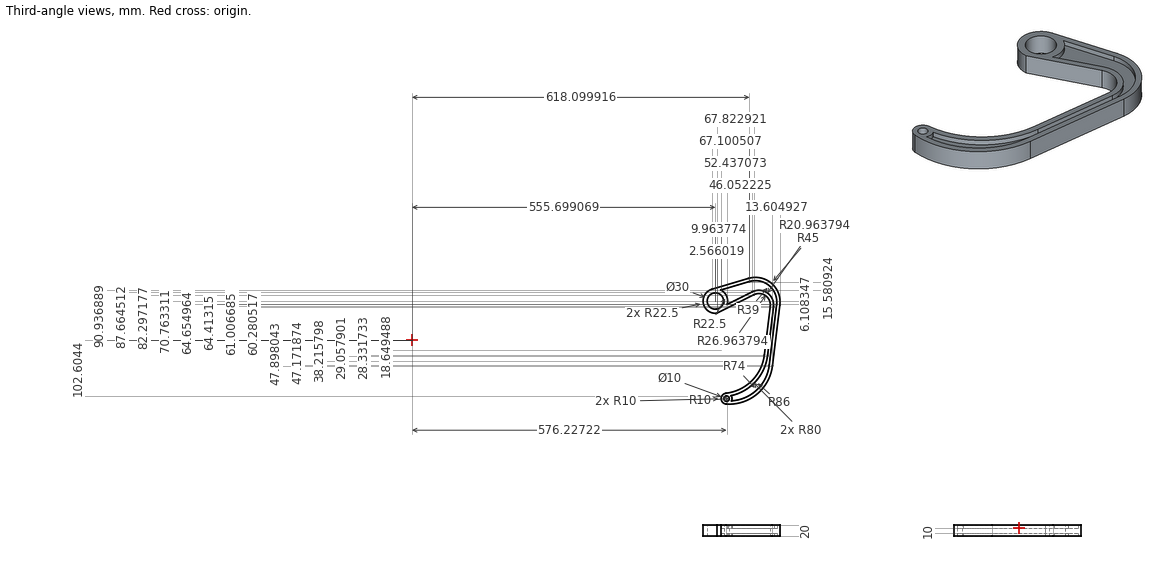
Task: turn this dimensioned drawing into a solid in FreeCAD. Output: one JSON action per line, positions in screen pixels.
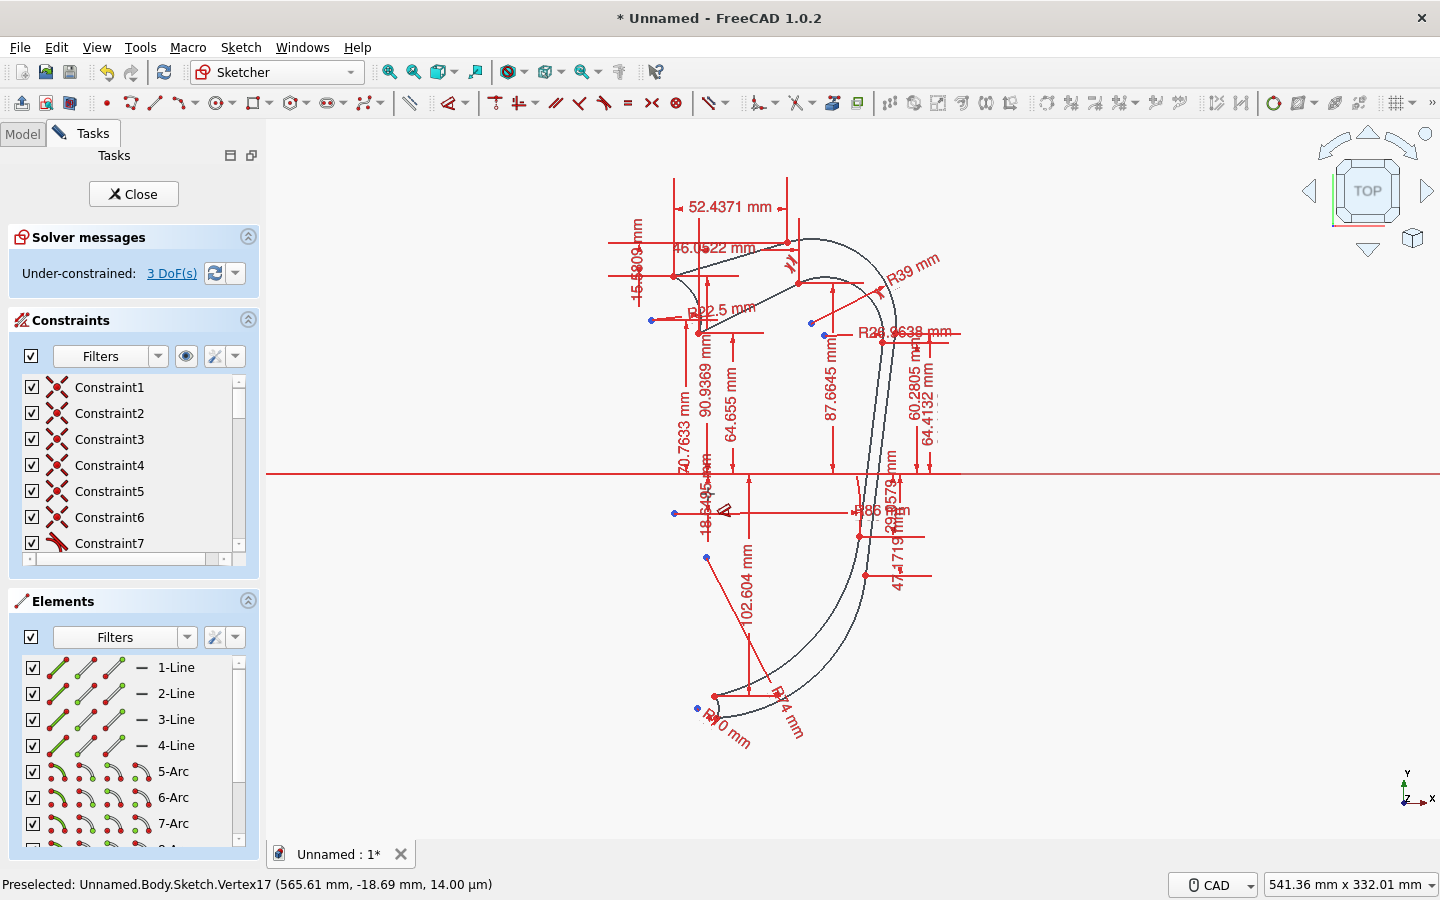
{"action": "left_click", "coordinate": [697, 709]}
{"action": "left_click", "coordinate": [496, 743]}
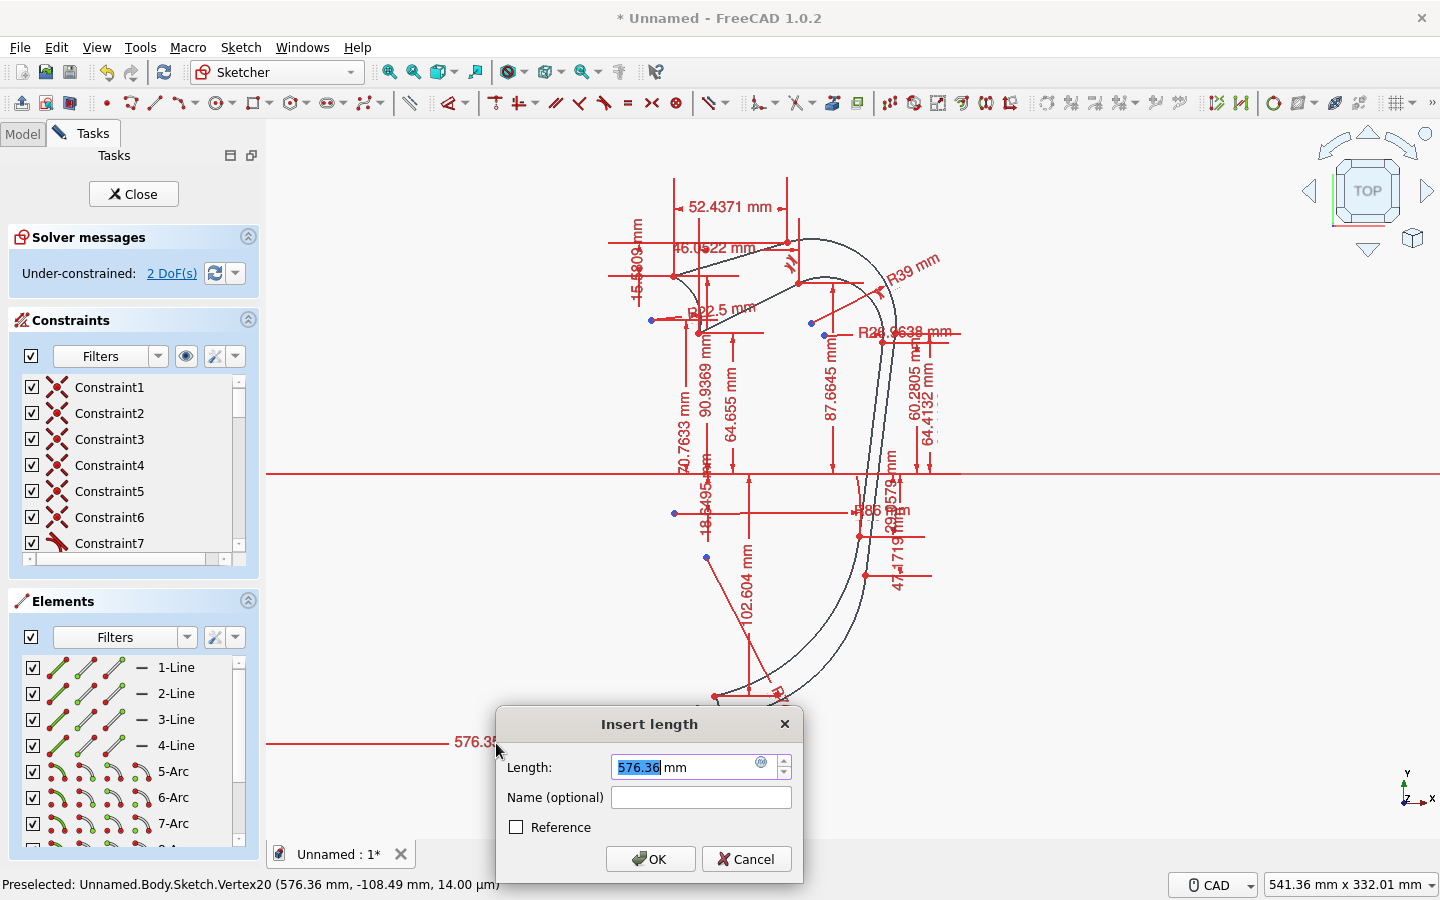
{"action": "type", "text": "576.22722"}
{"action": "key", "text": "Return"}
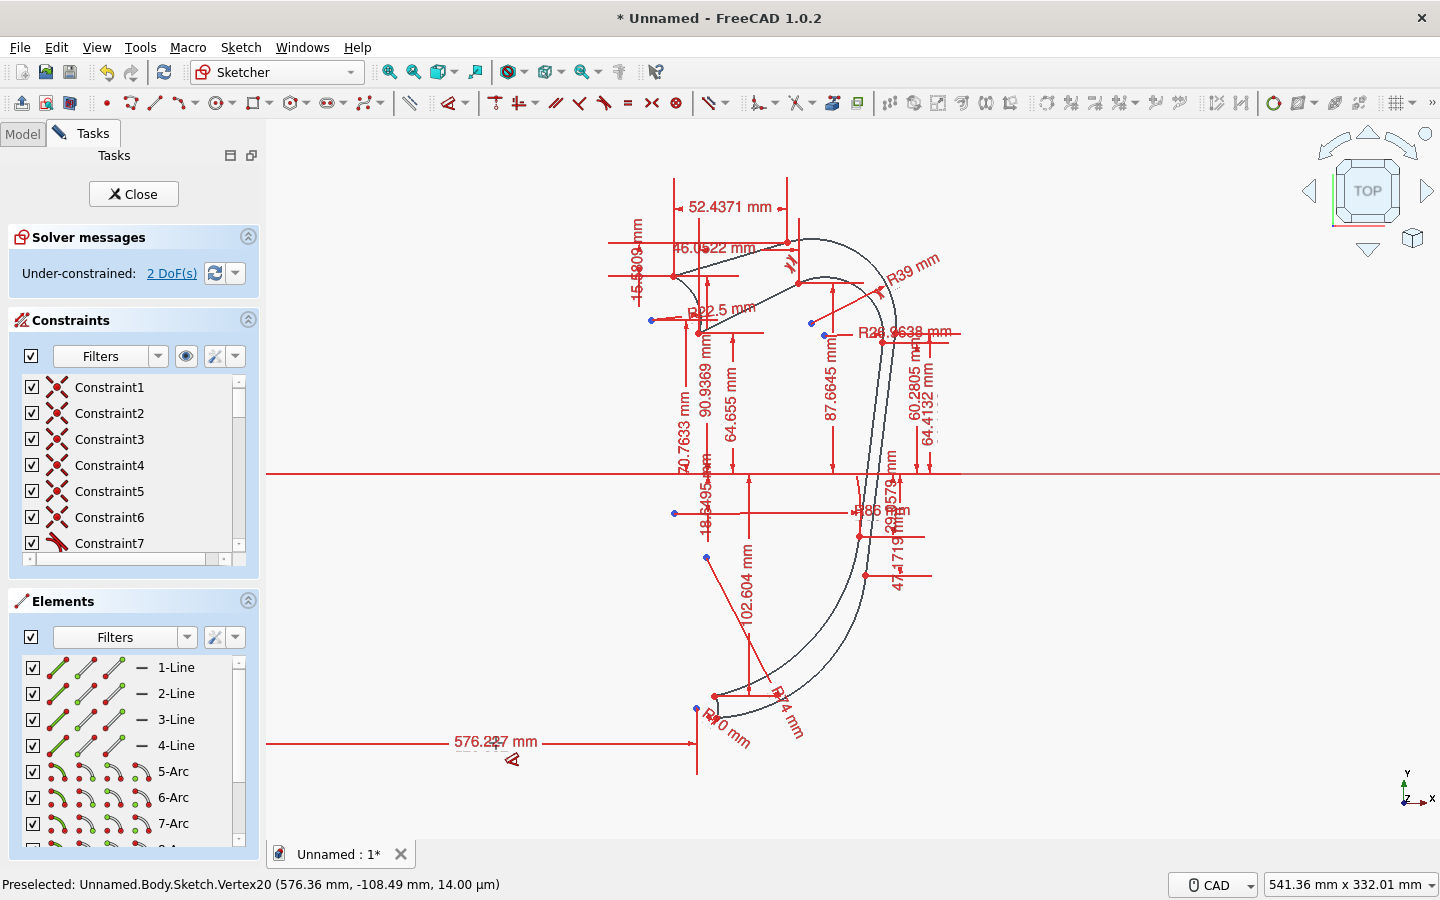
{"action": "left_click", "coordinate": [706, 558]}
{"action": "left_click", "coordinate": [740, 516]}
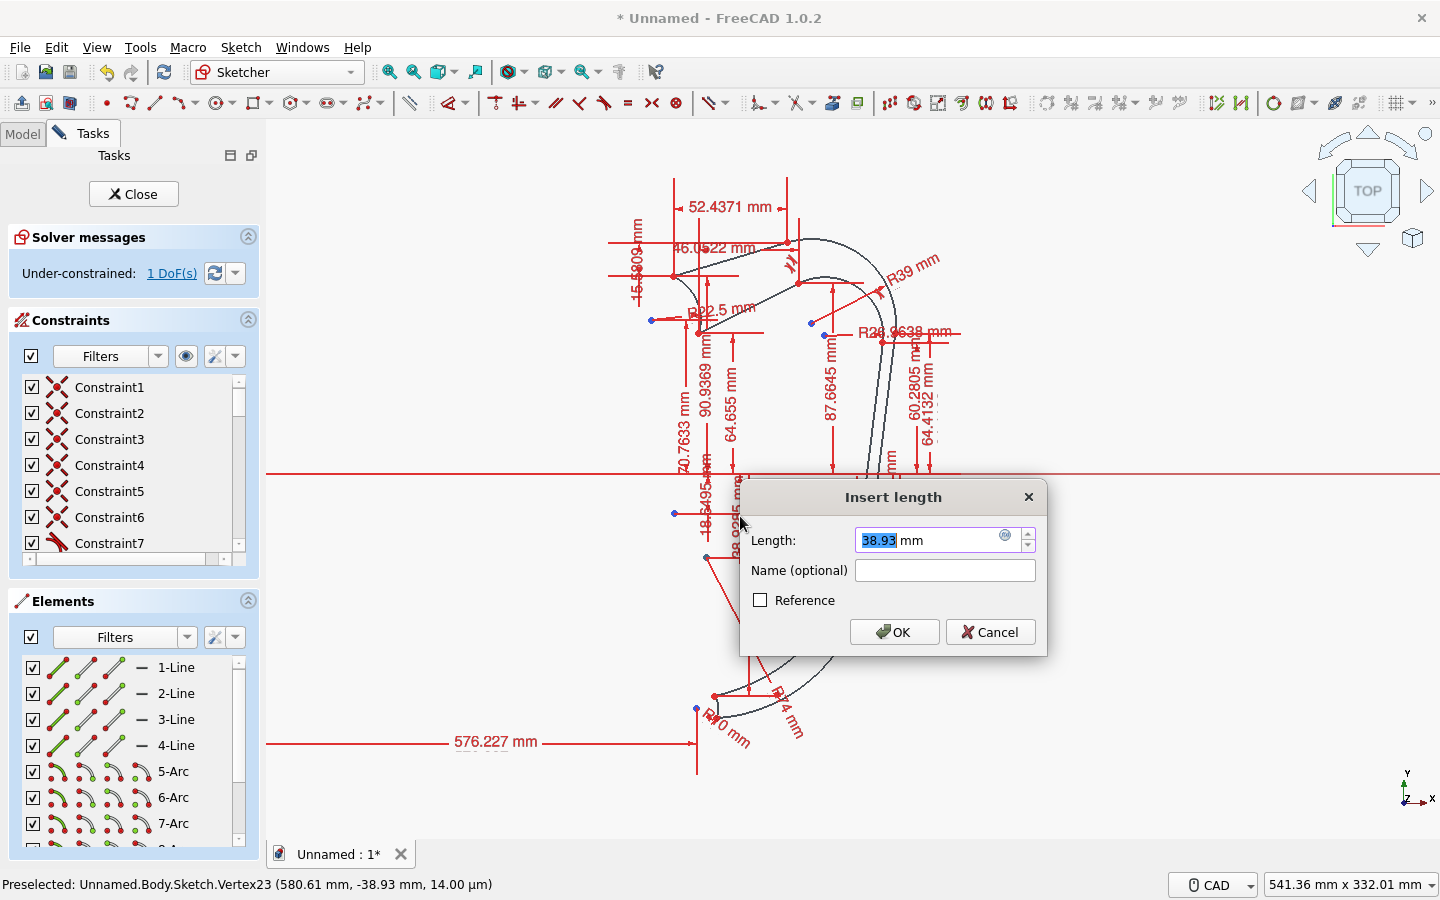
{"action": "type", "text": "38.215798"}
{"action": "key", "text": "Return"}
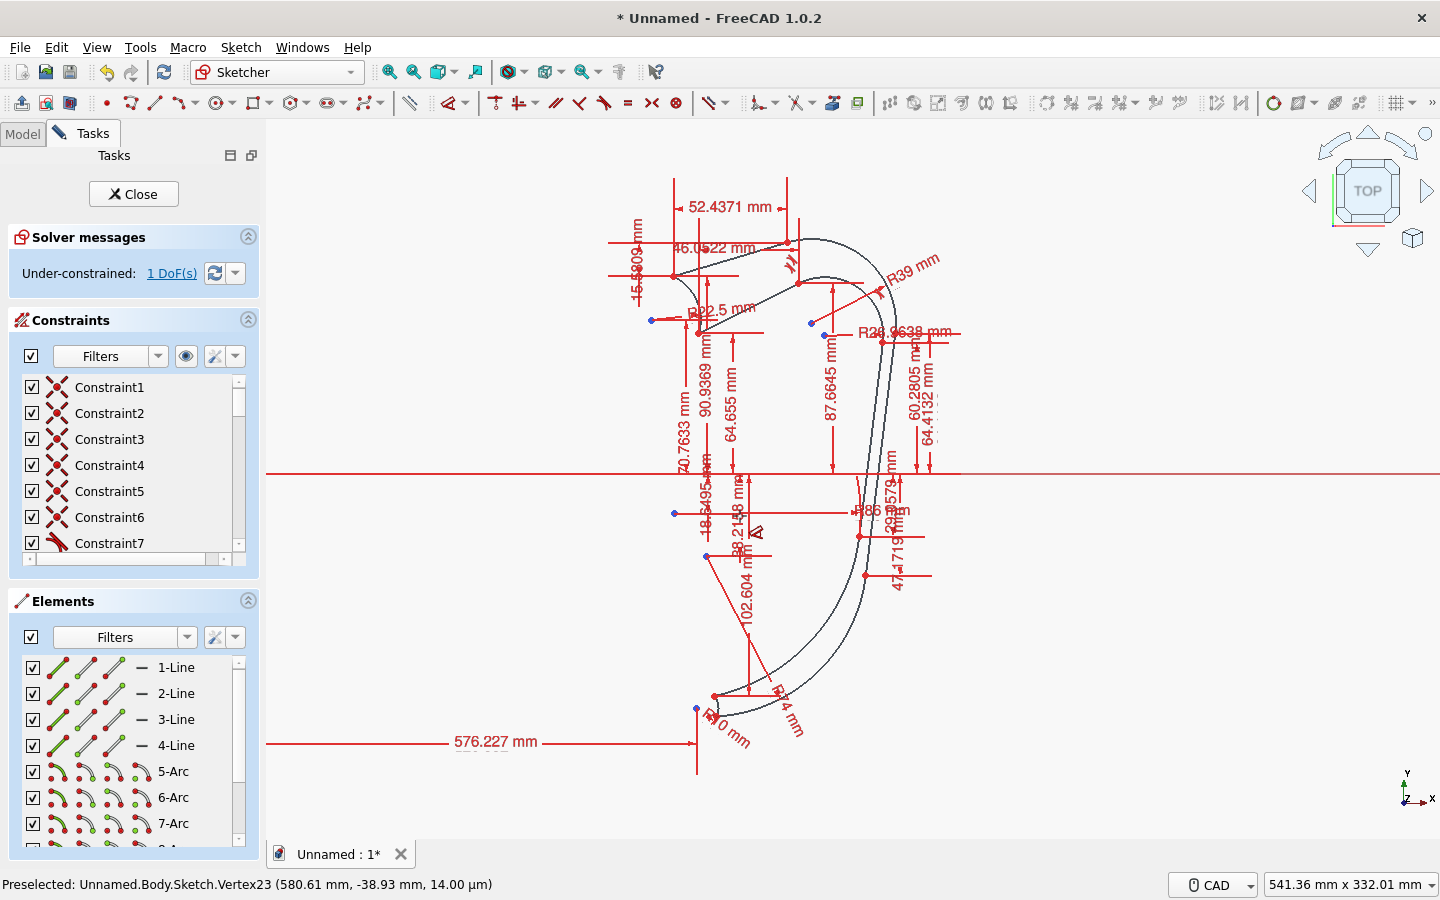
{"action": "left_click", "coordinate": [787, 243]}
{"action": "left_click", "coordinate": [541, 209]}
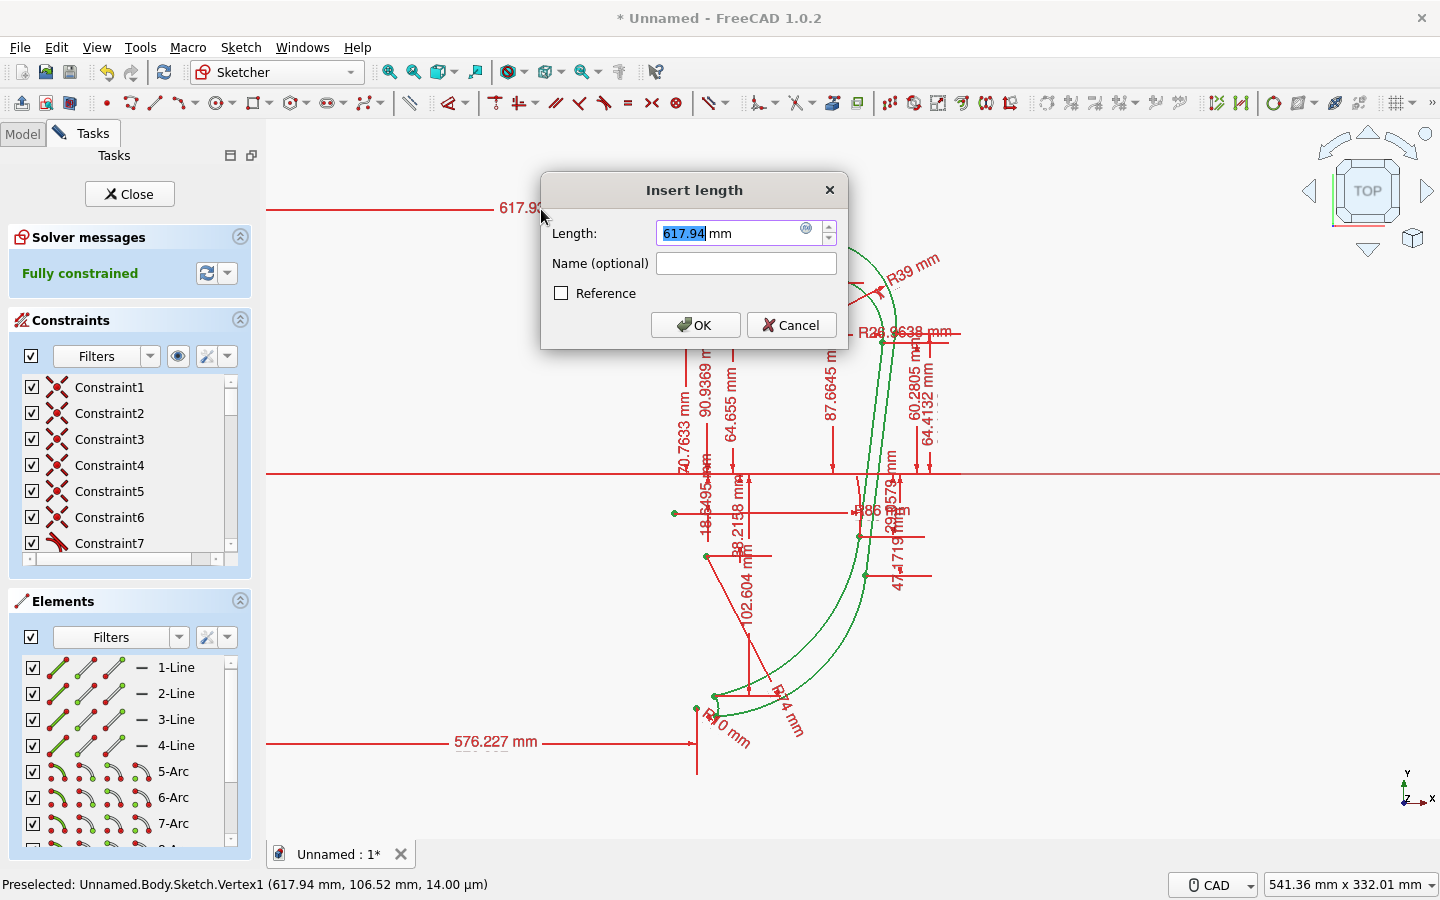
{"action": "type", "text": "618.099916"}
{"action": "key", "text": "Return"}
{"action": "key", "text": "Escape"}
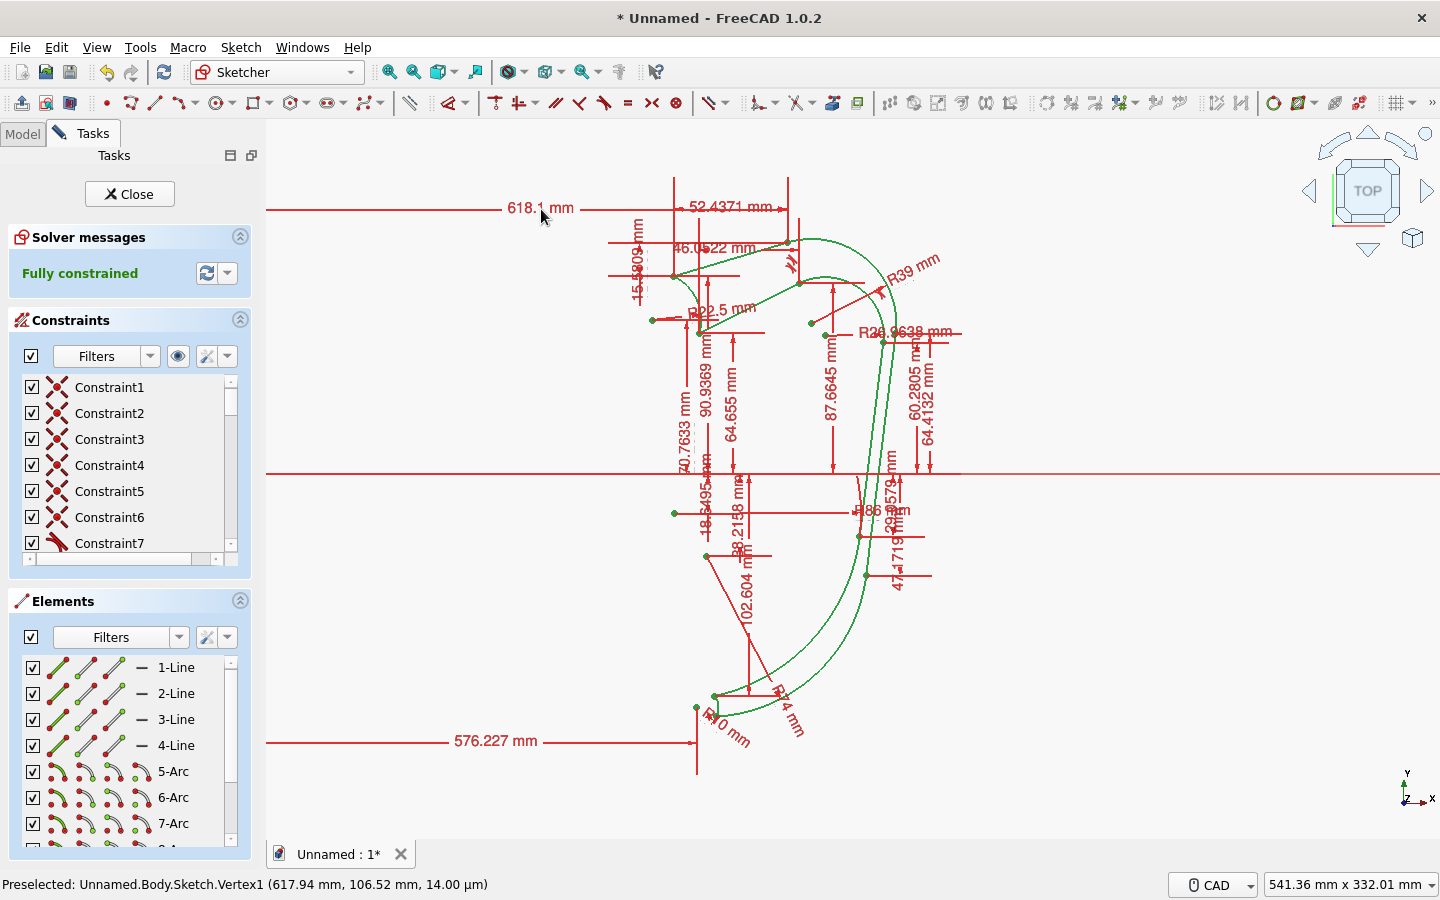
{"action": "left_click", "coordinate": [130, 194]}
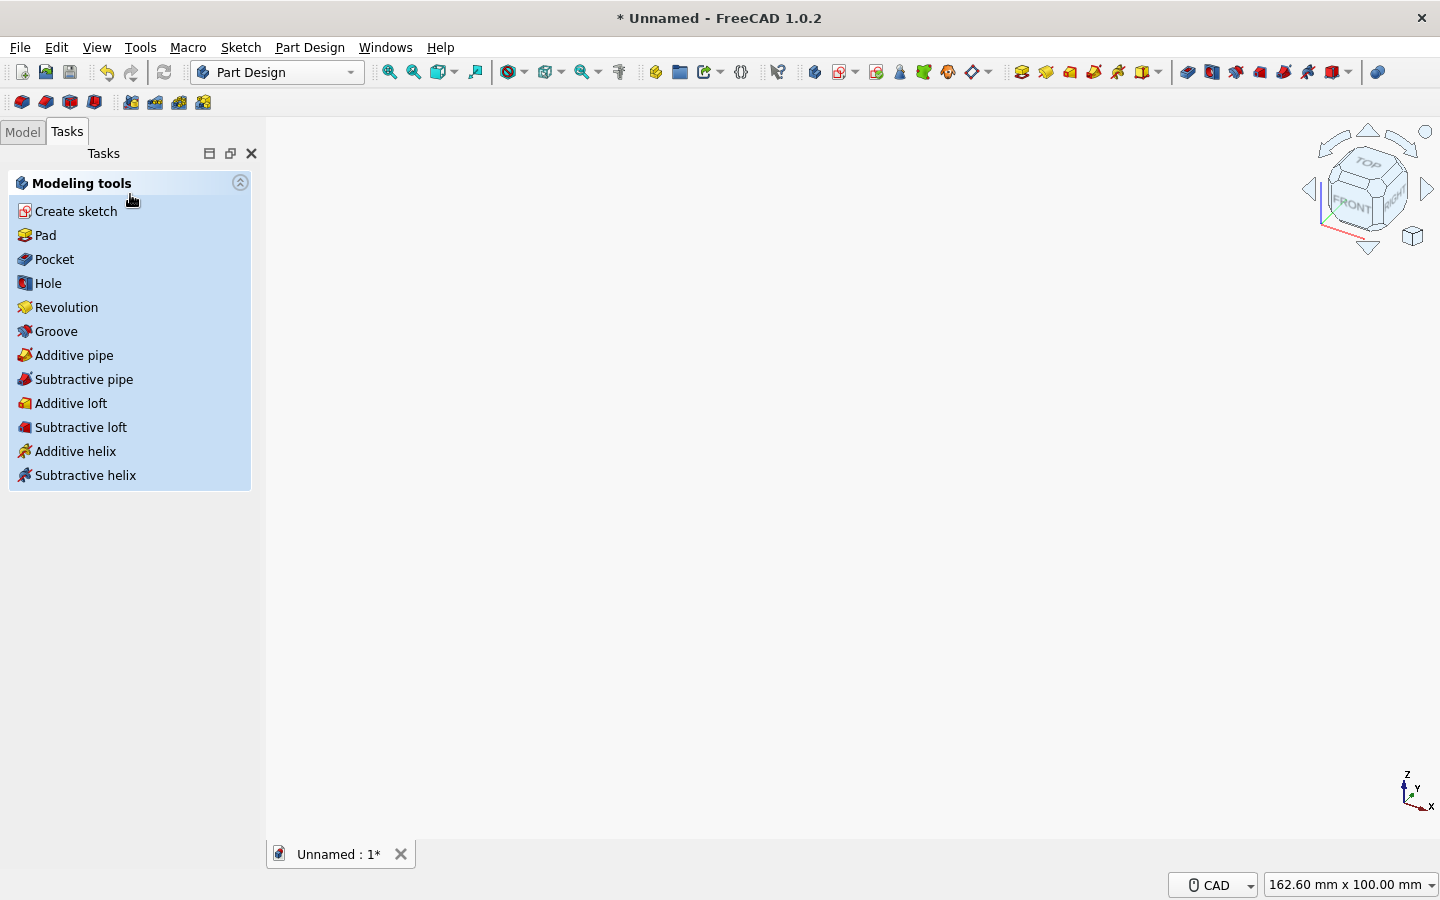
{"action": "left_click", "coordinate": [1022, 72]}